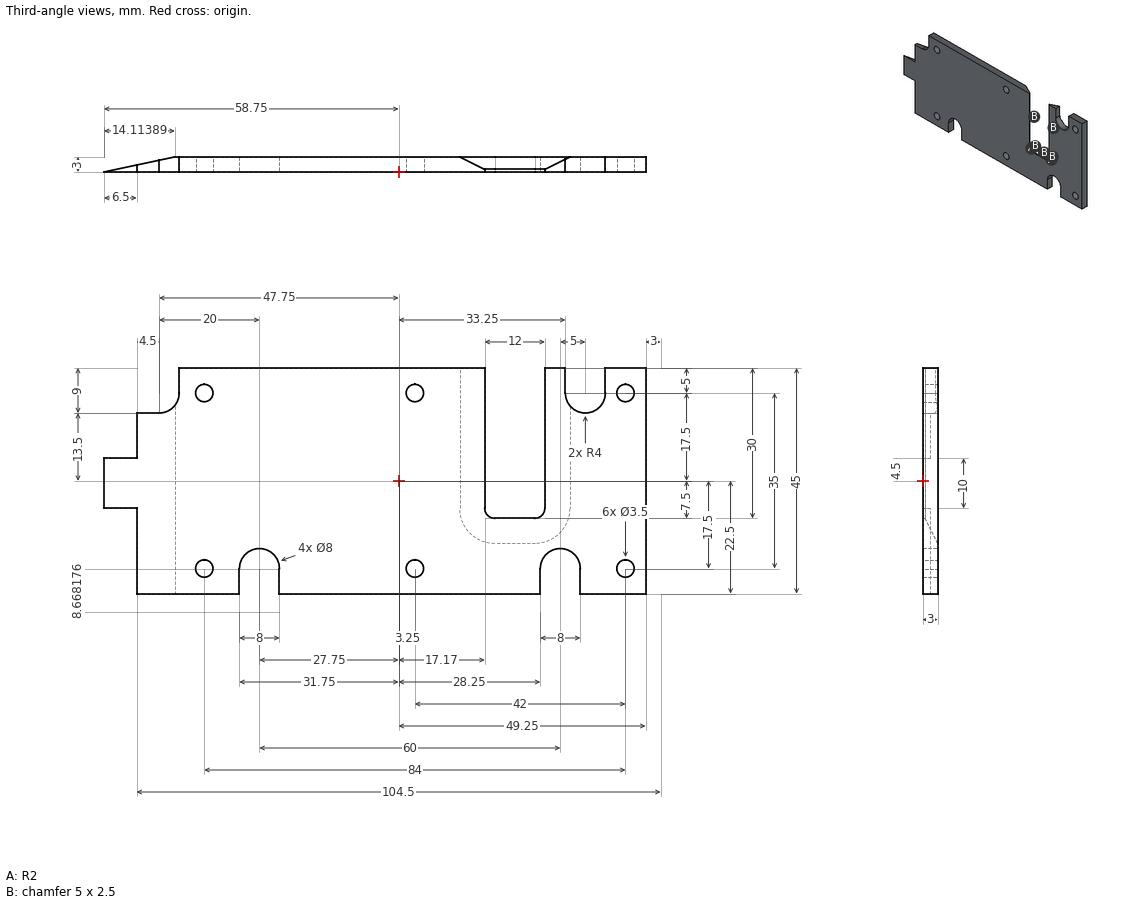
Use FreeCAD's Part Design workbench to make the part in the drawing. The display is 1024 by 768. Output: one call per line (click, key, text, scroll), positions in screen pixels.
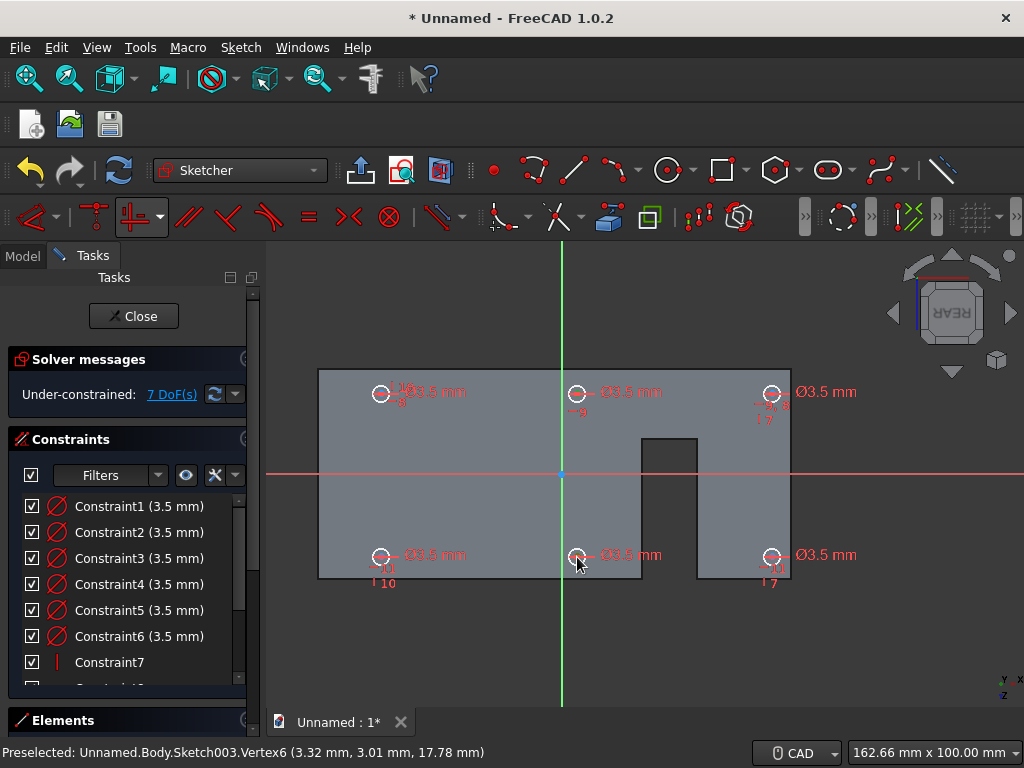
click(162, 218)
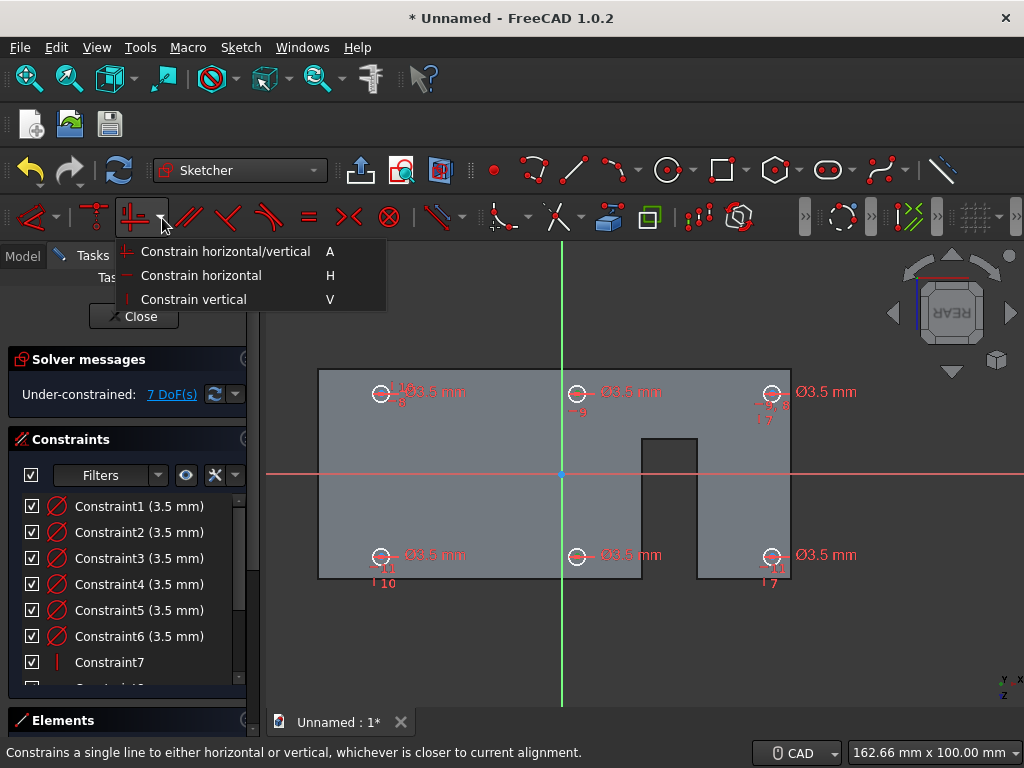
click(251, 299)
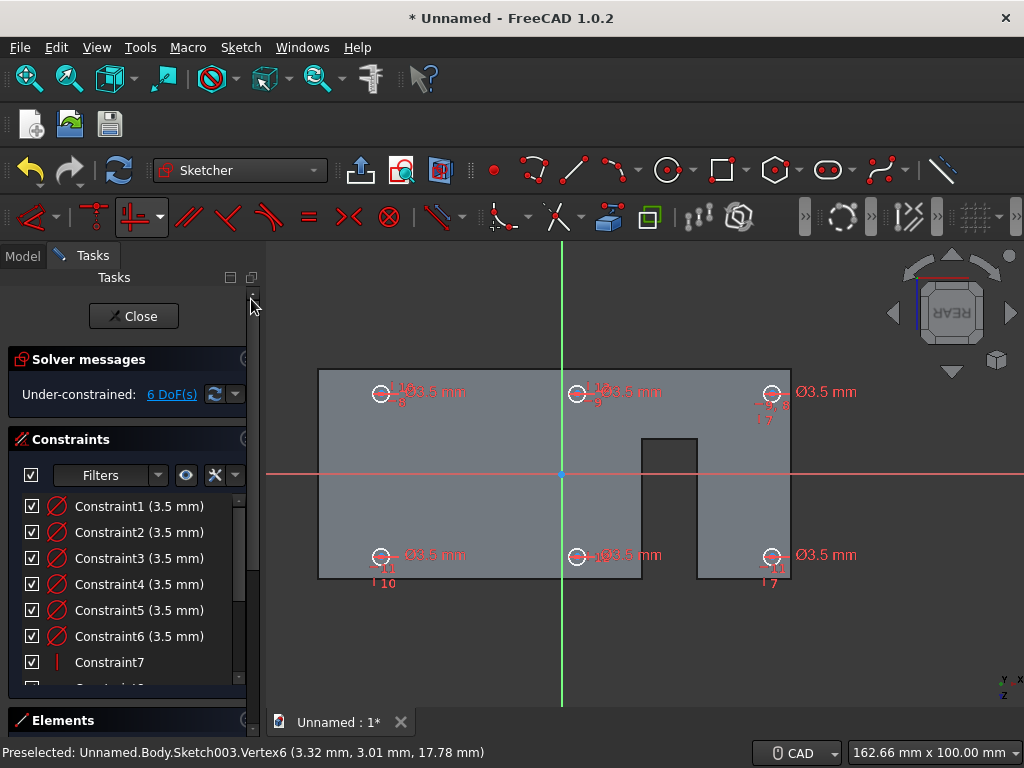
click(772, 557)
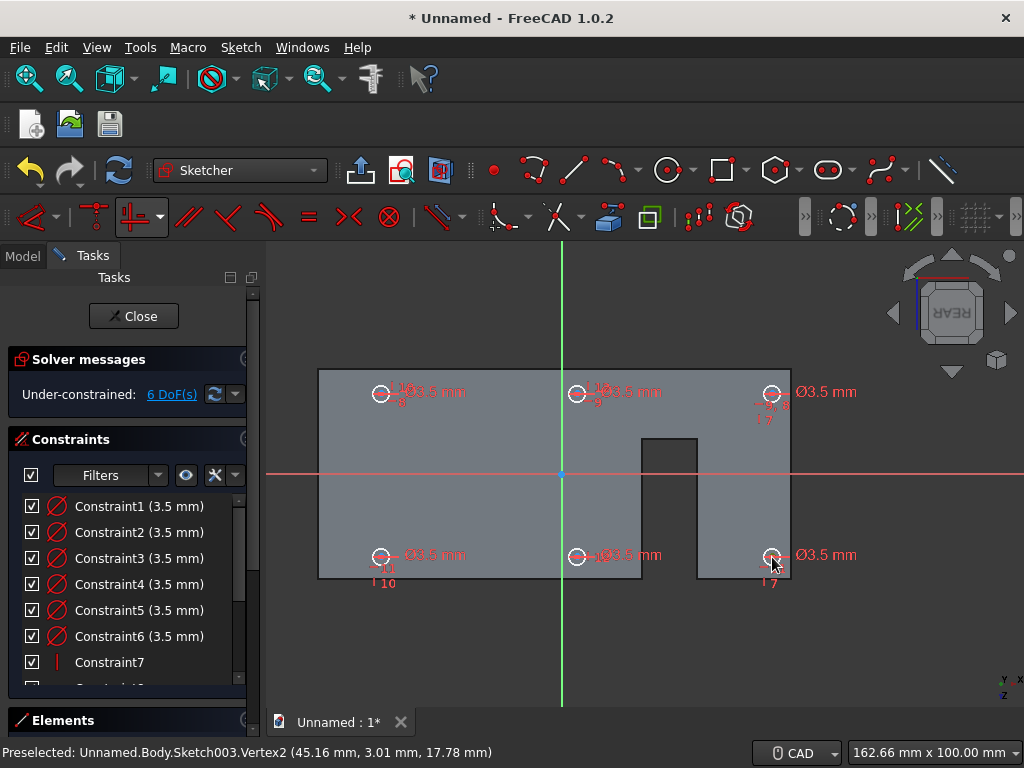
click(577, 557)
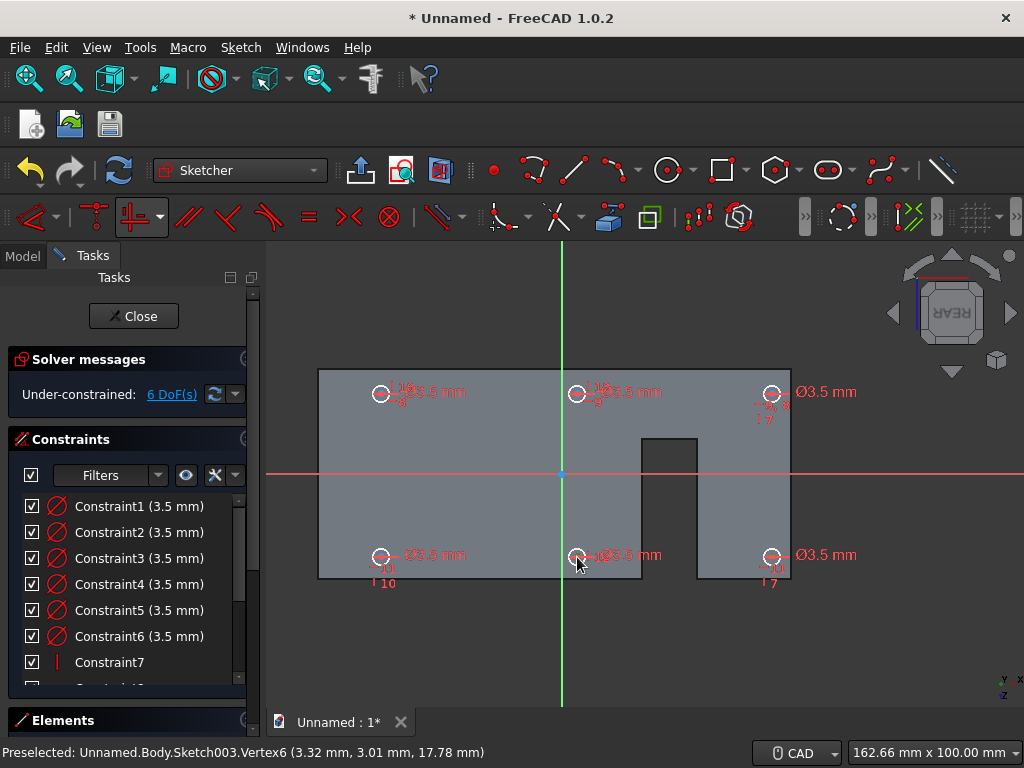
key(h)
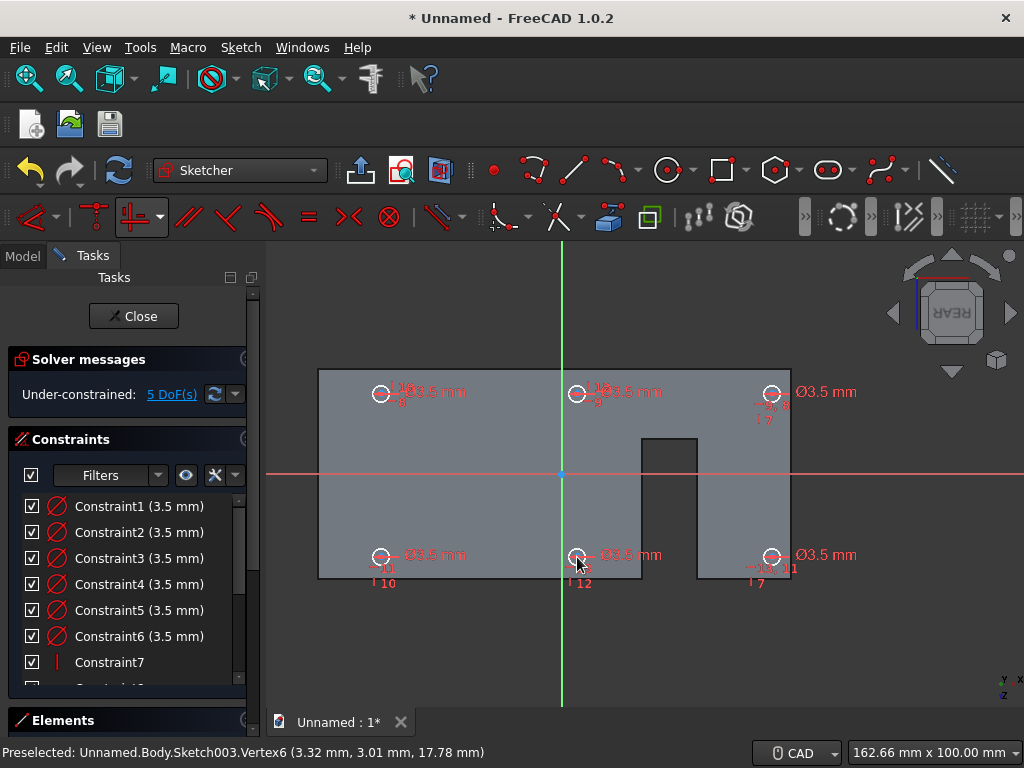
click(32, 218)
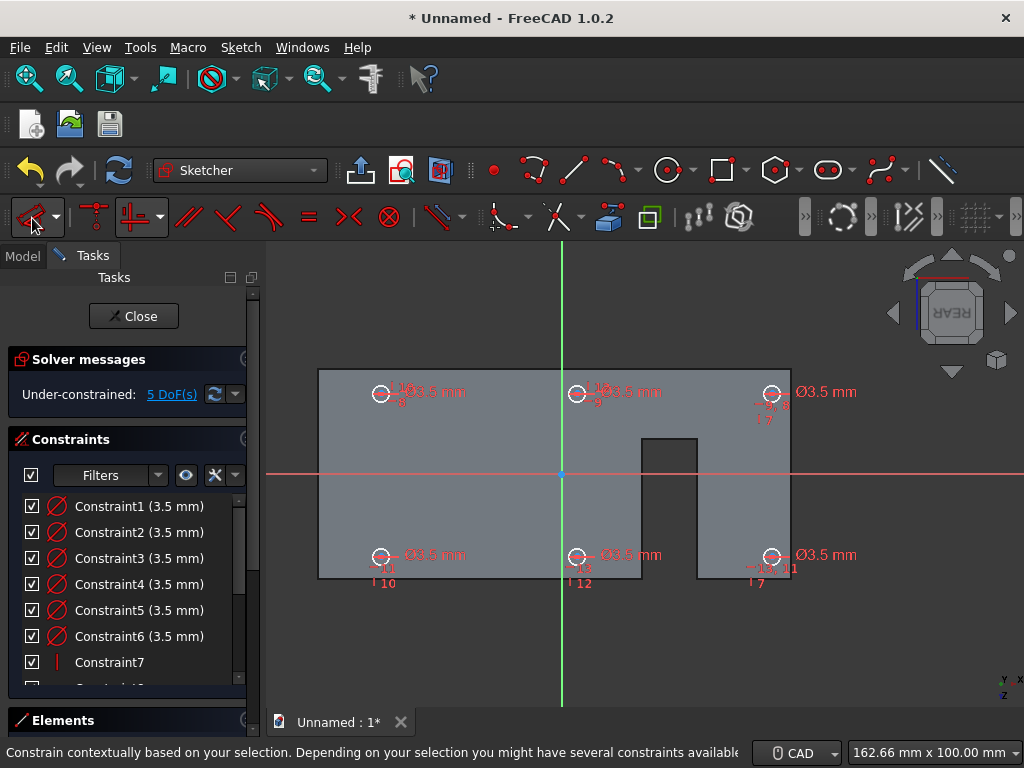
click(772, 394)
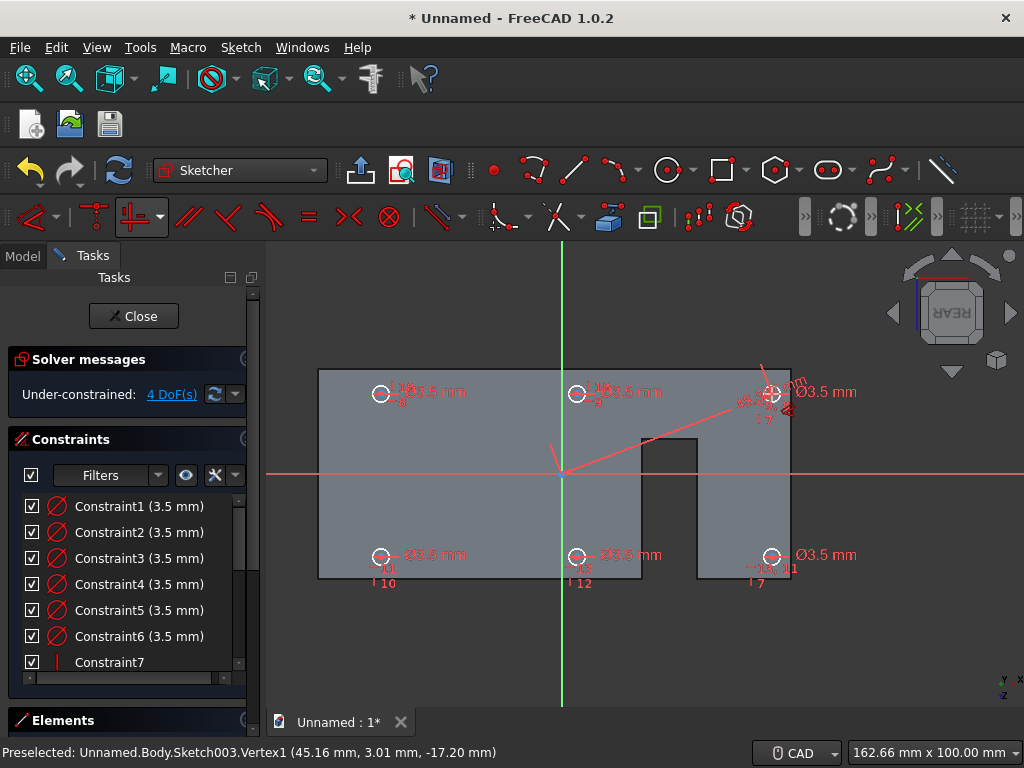
click(772, 557)
click(806, 438)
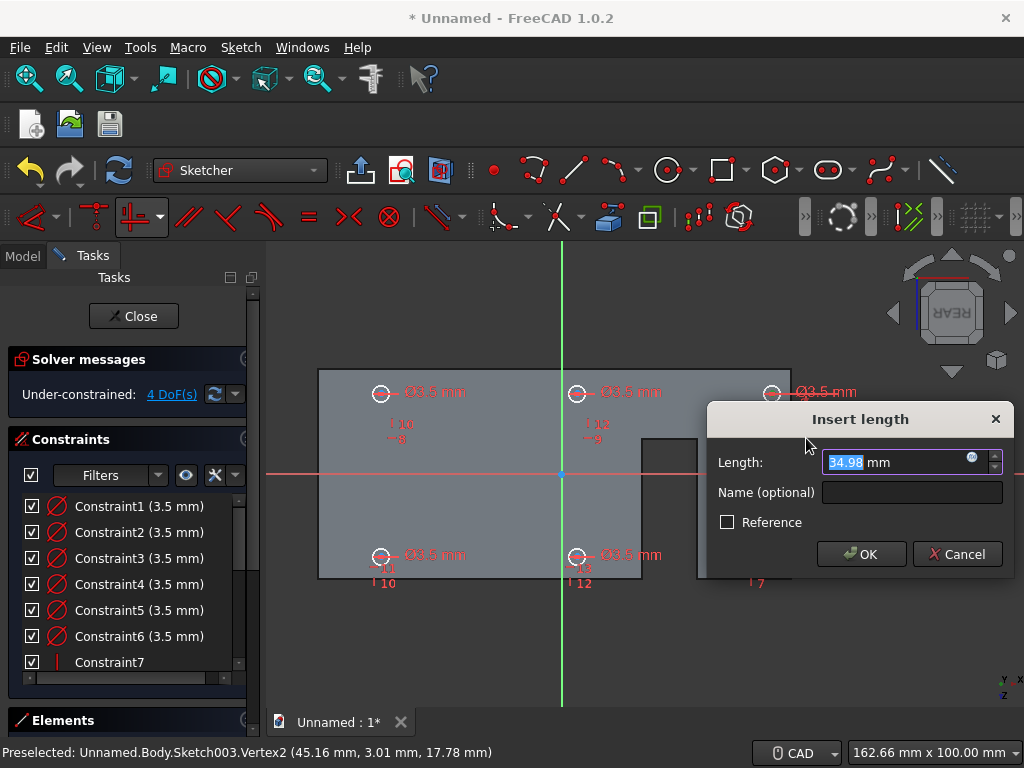
text(35)
key(Return)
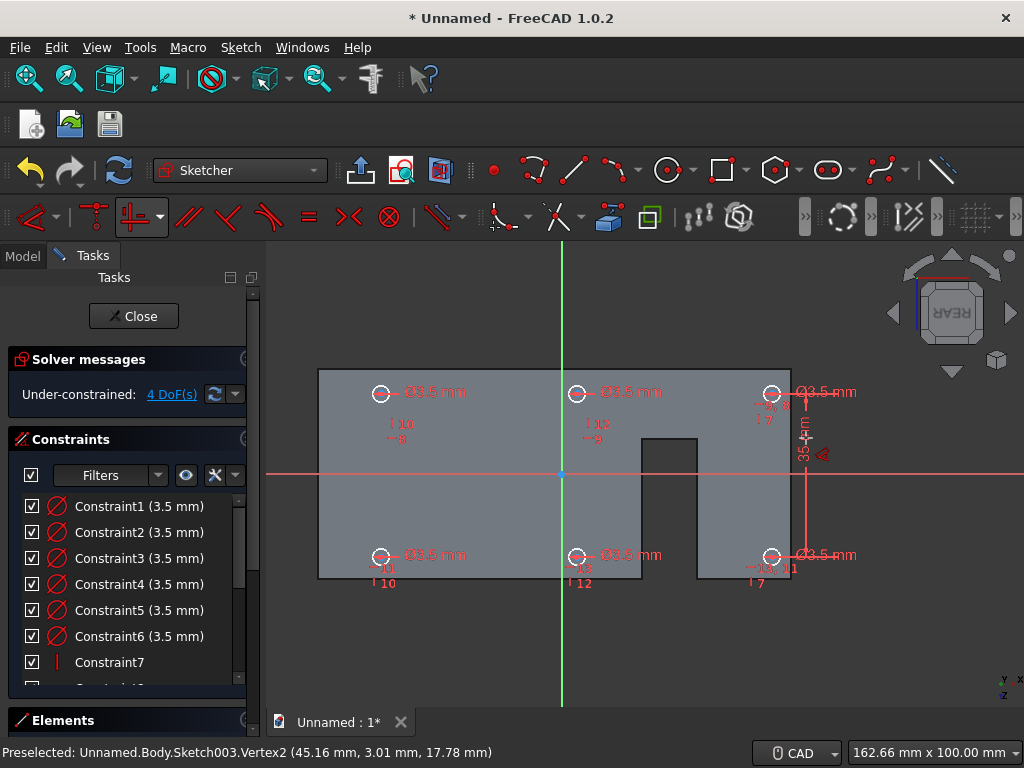
click(772, 394)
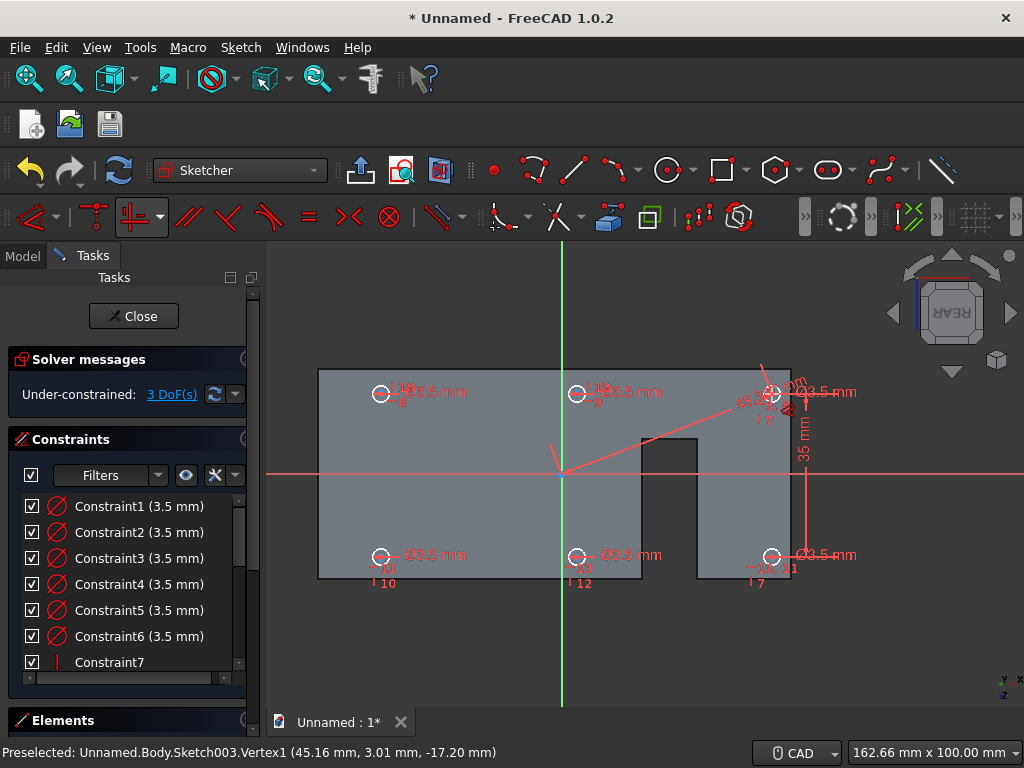
click(381, 394)
click(577, 360)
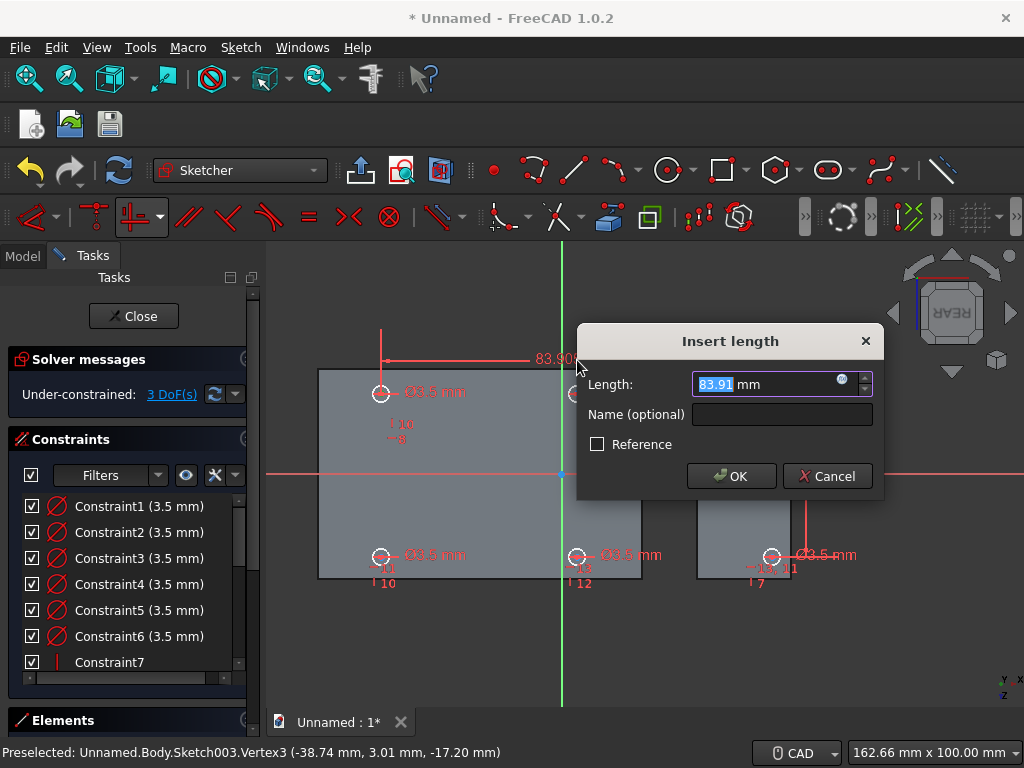
text(84)
key(Return)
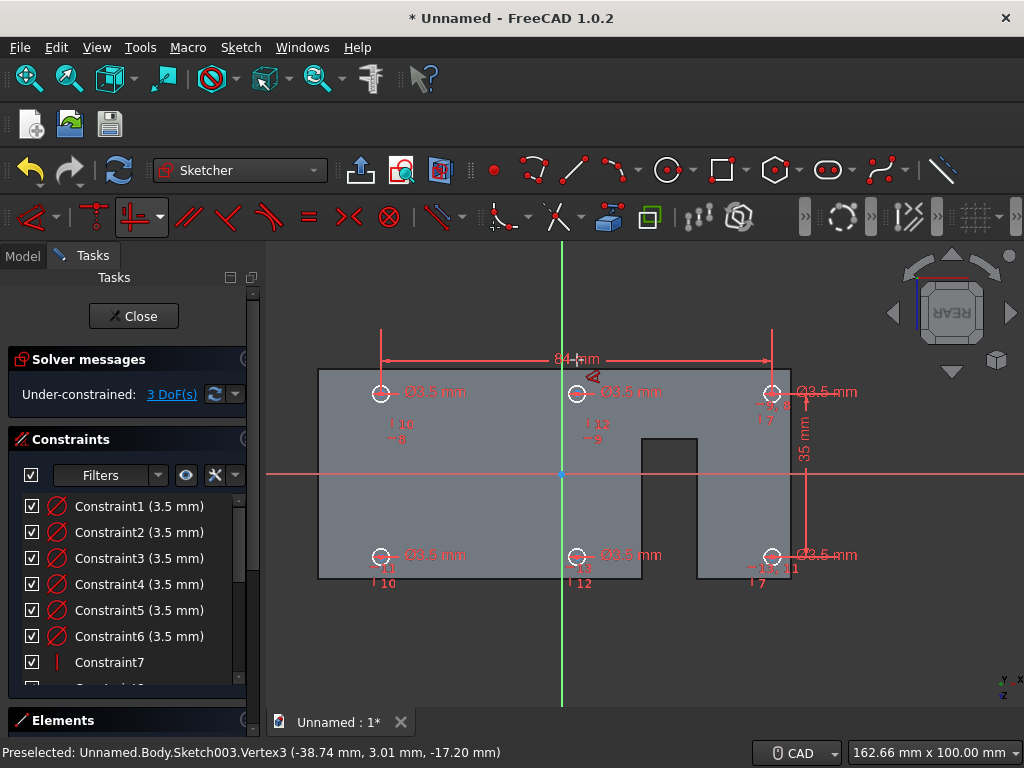
click(772, 394)